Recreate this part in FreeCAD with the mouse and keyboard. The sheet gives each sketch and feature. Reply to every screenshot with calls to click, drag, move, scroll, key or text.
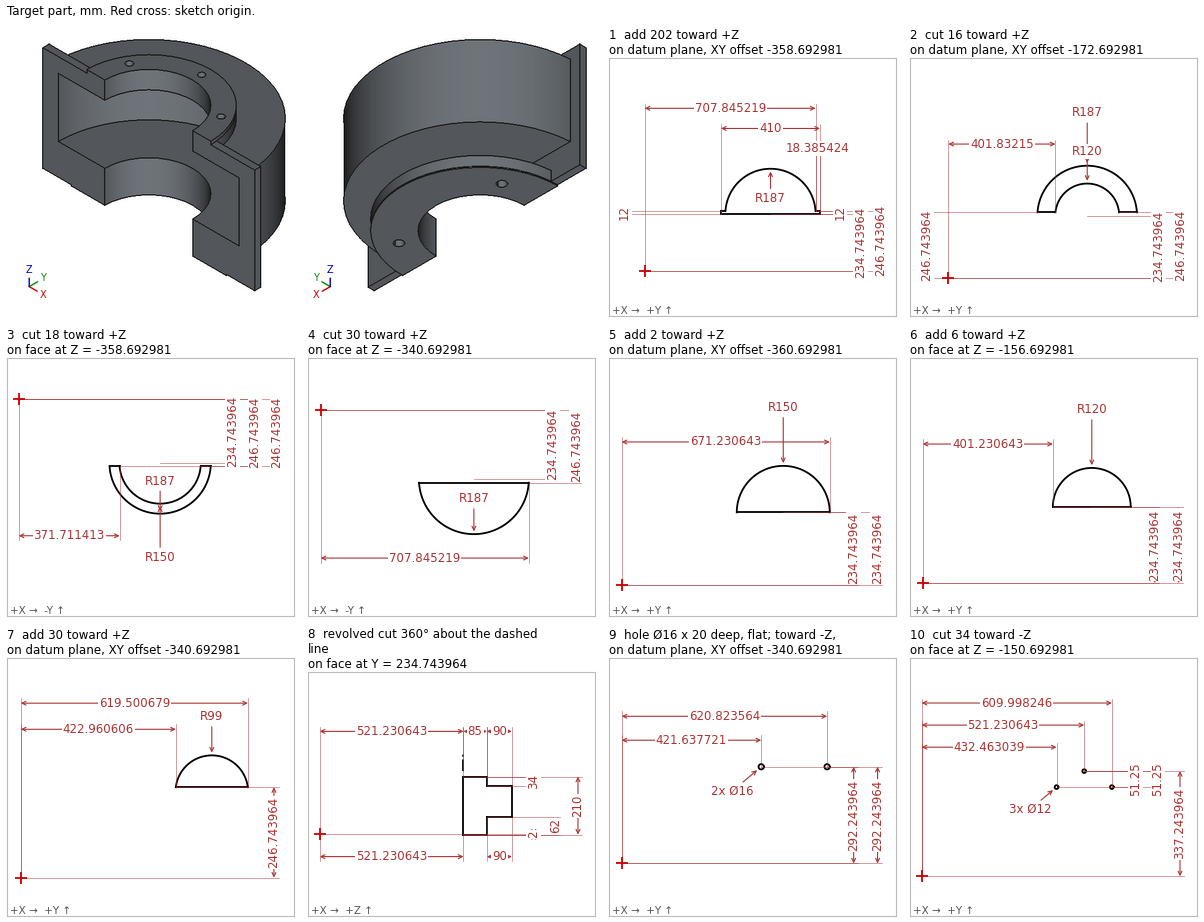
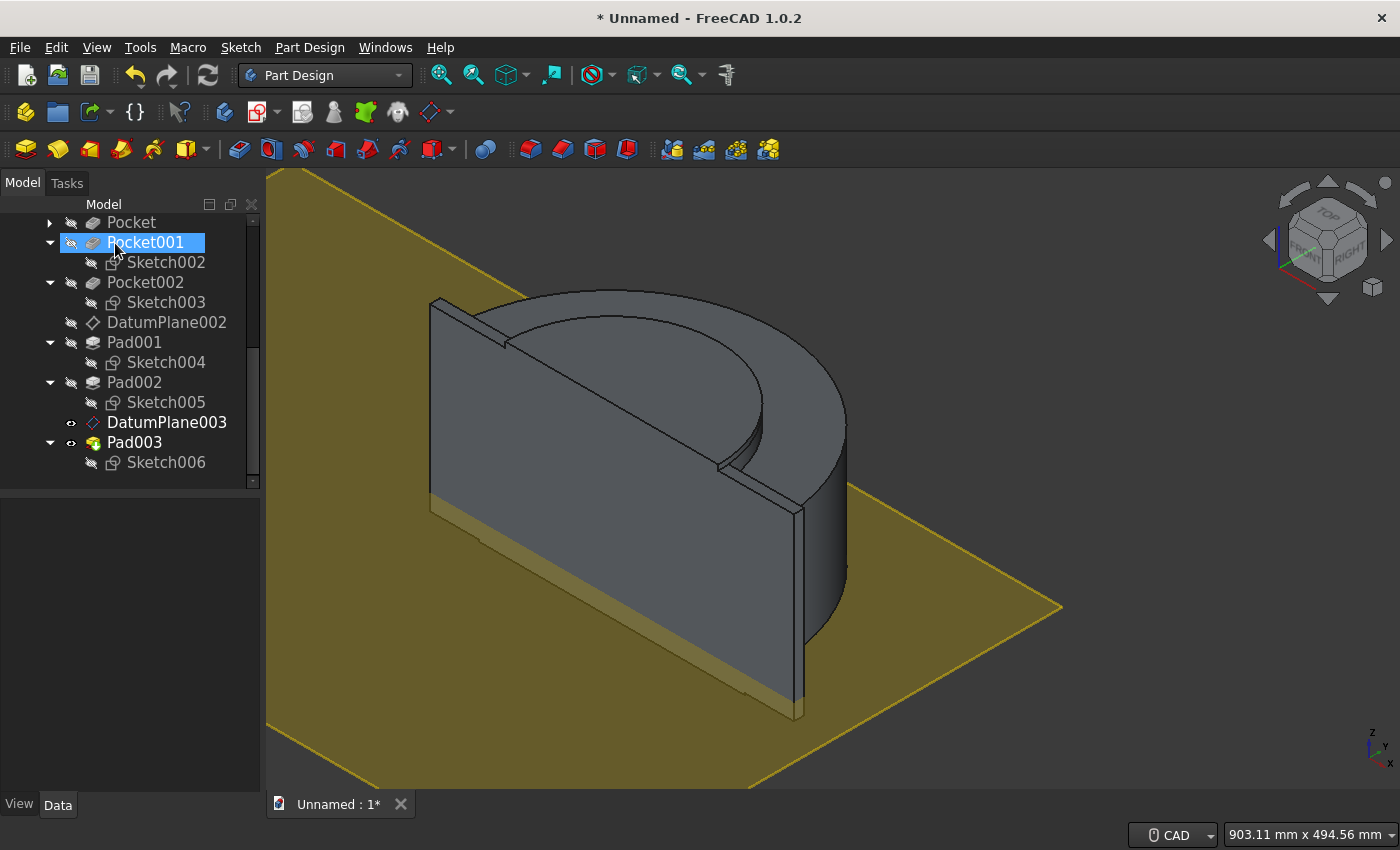
click(116, 423)
key(space)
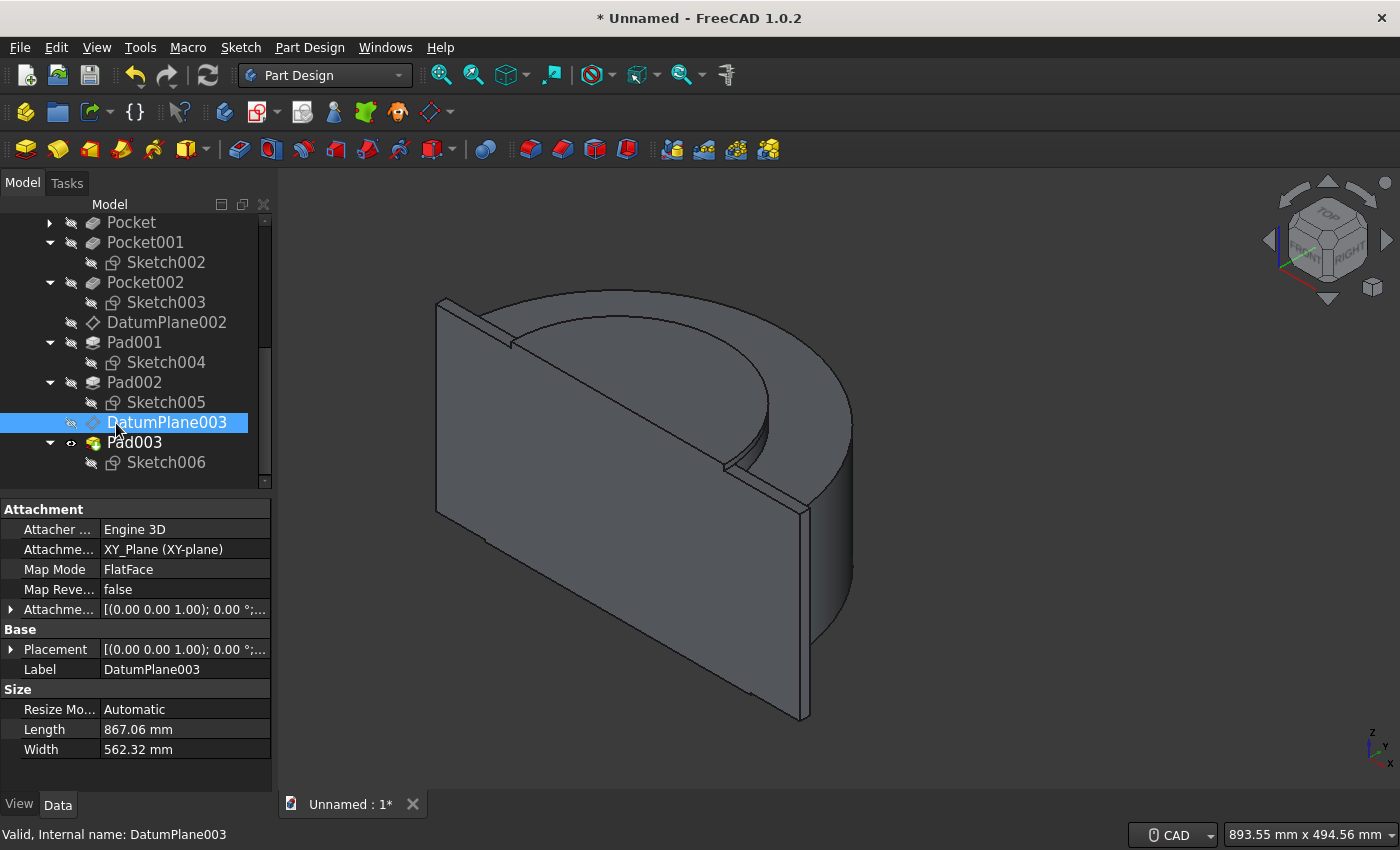
click(670, 540)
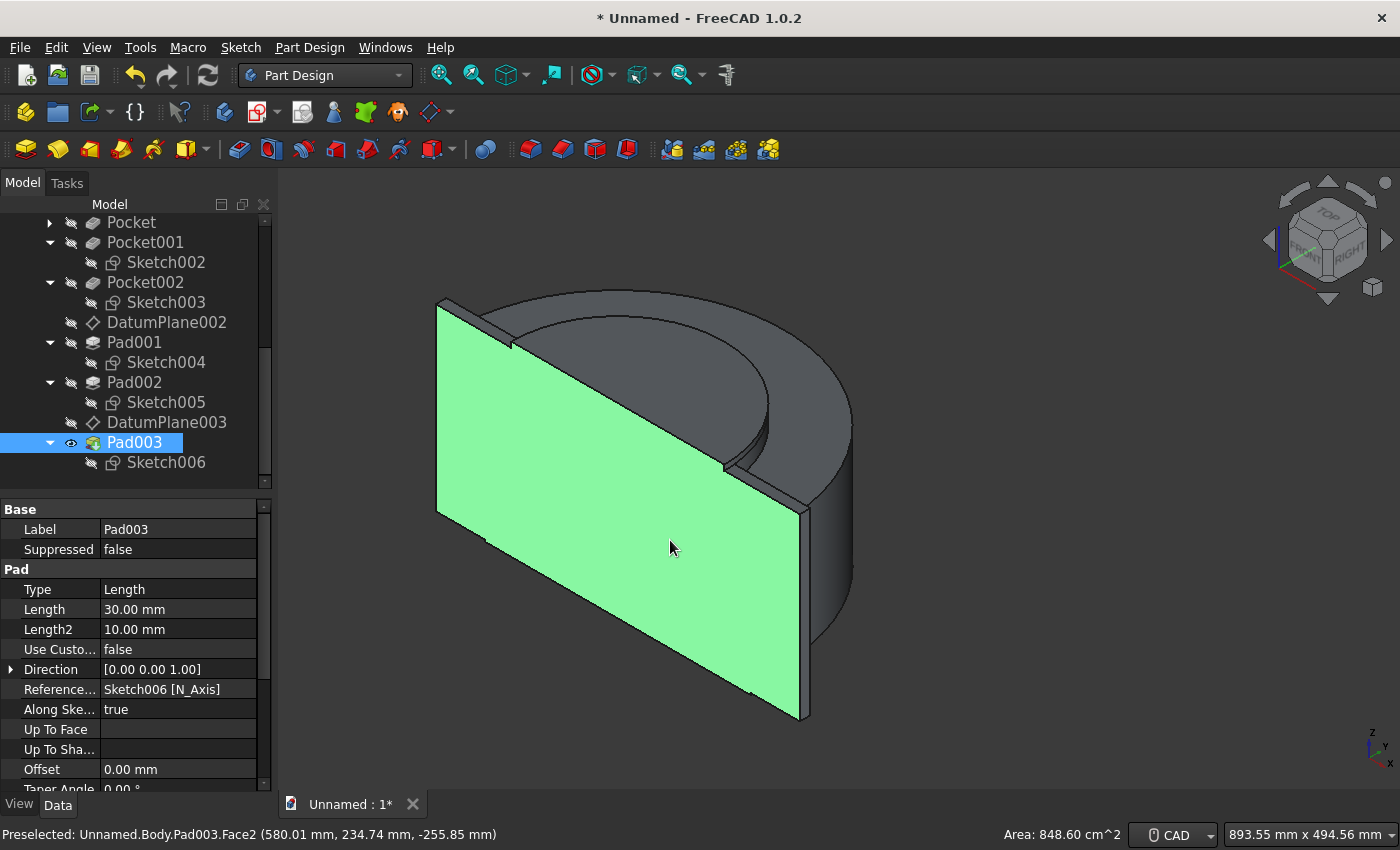
click(258, 112)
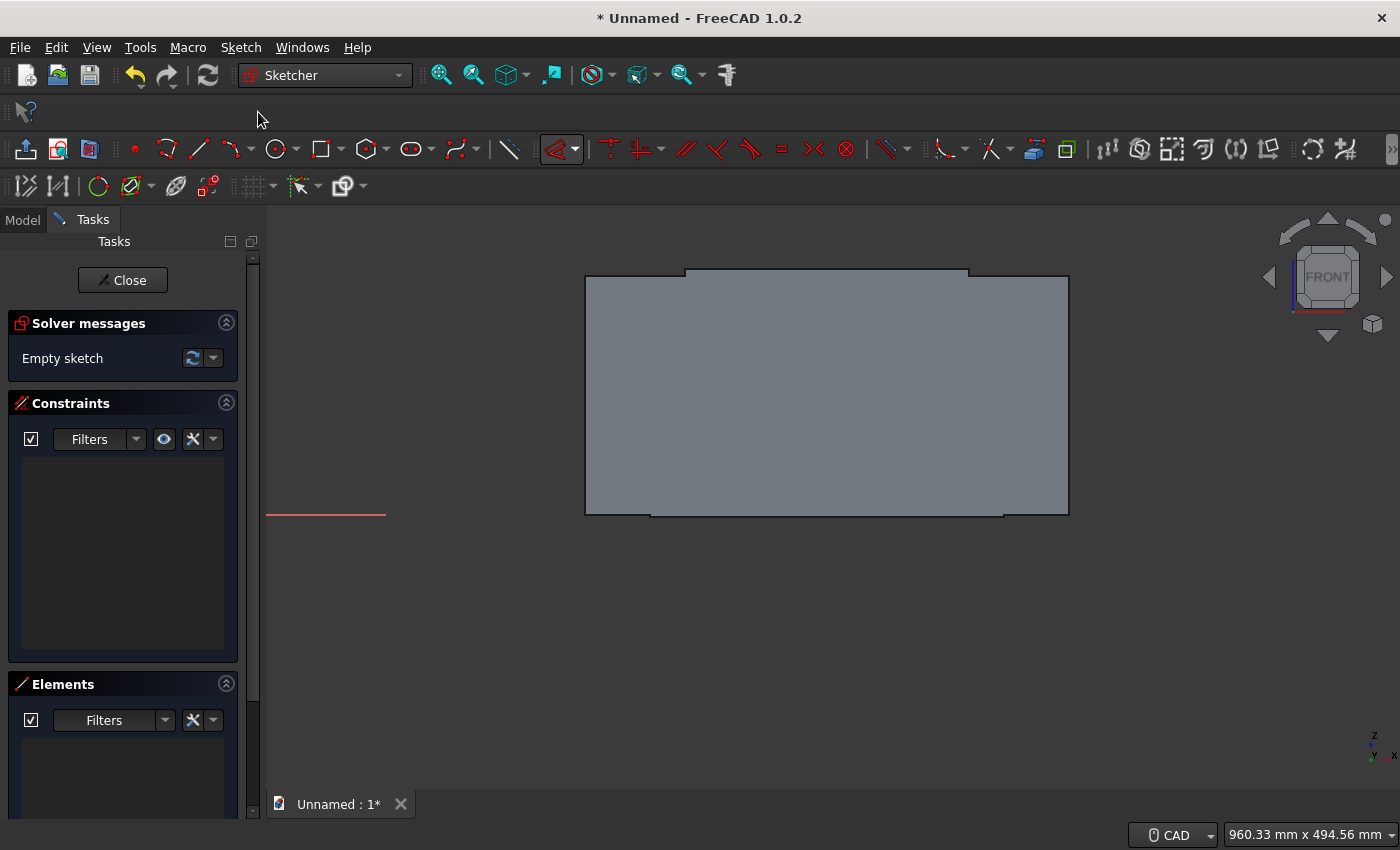
scroll(1235, 761, down, 1)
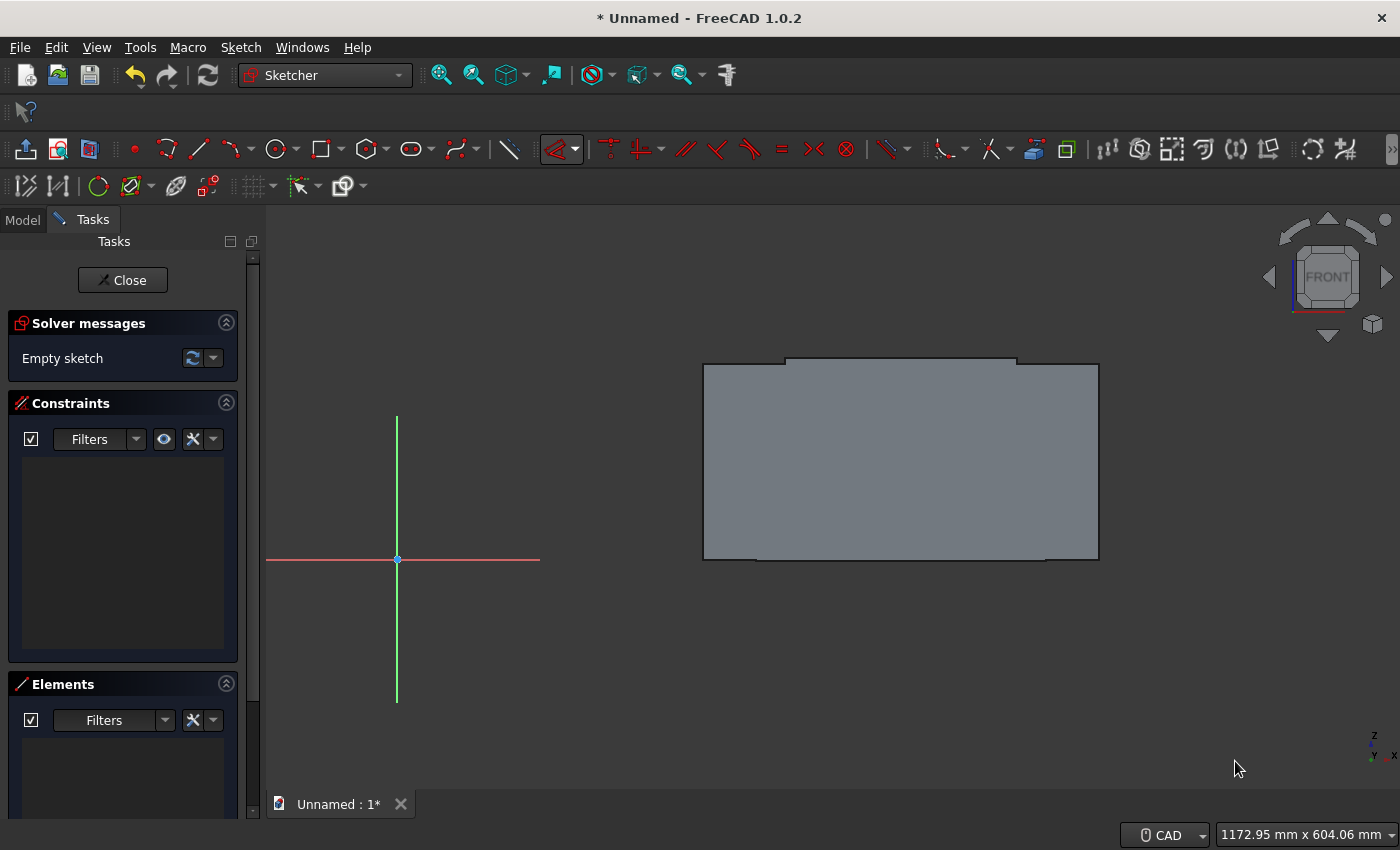
click(168, 150)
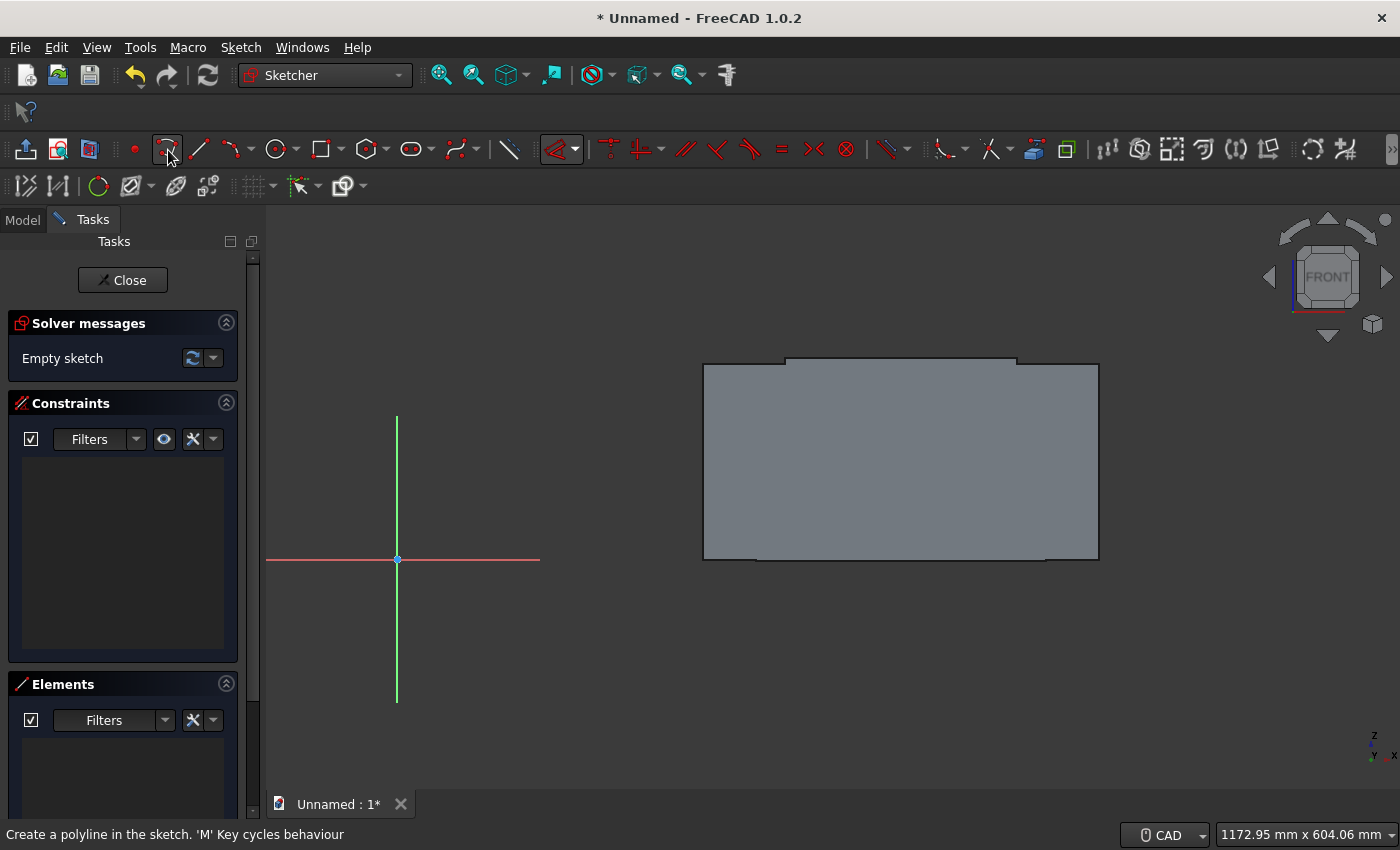
scroll(901, 561, up, 11)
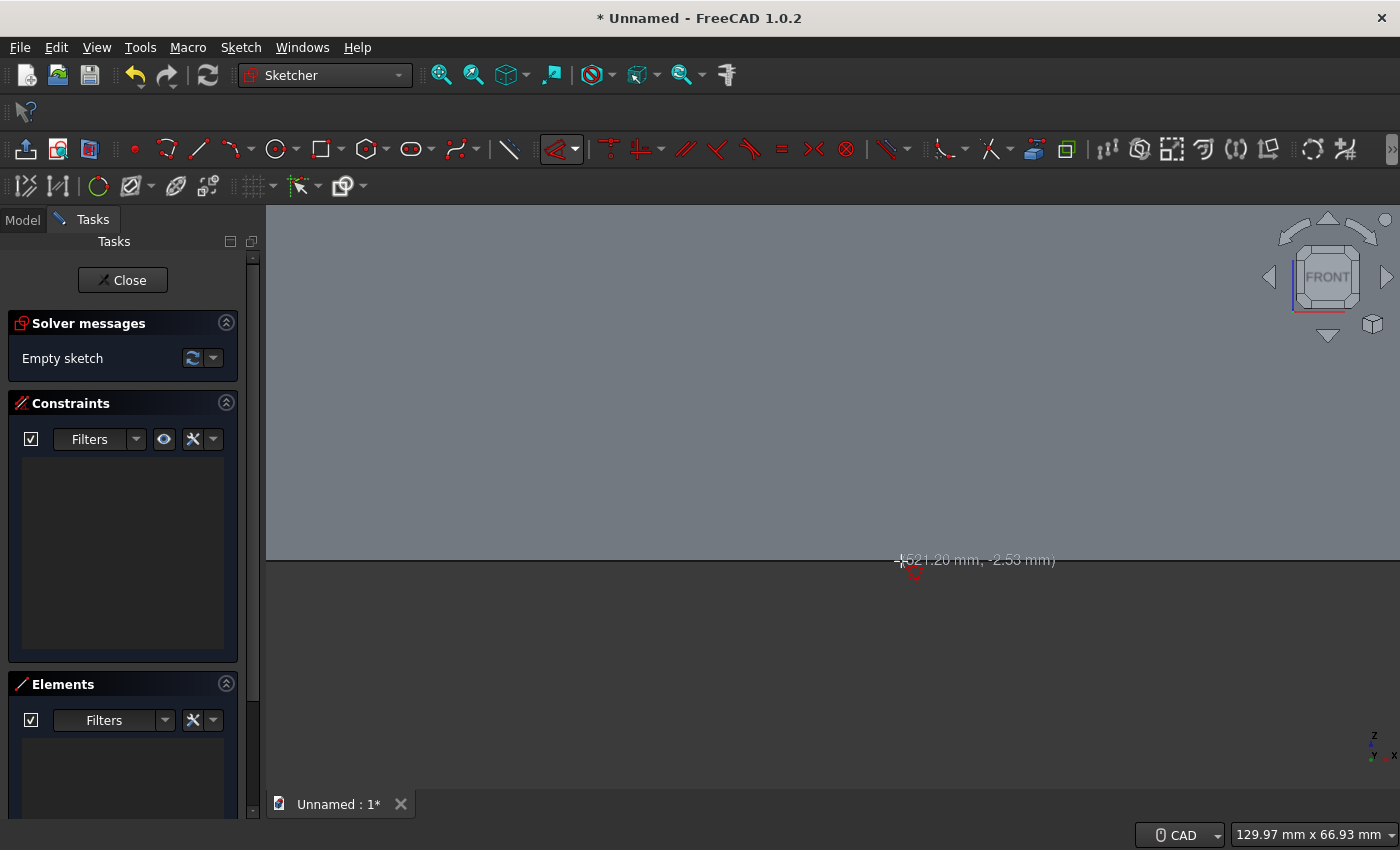
click(897, 561)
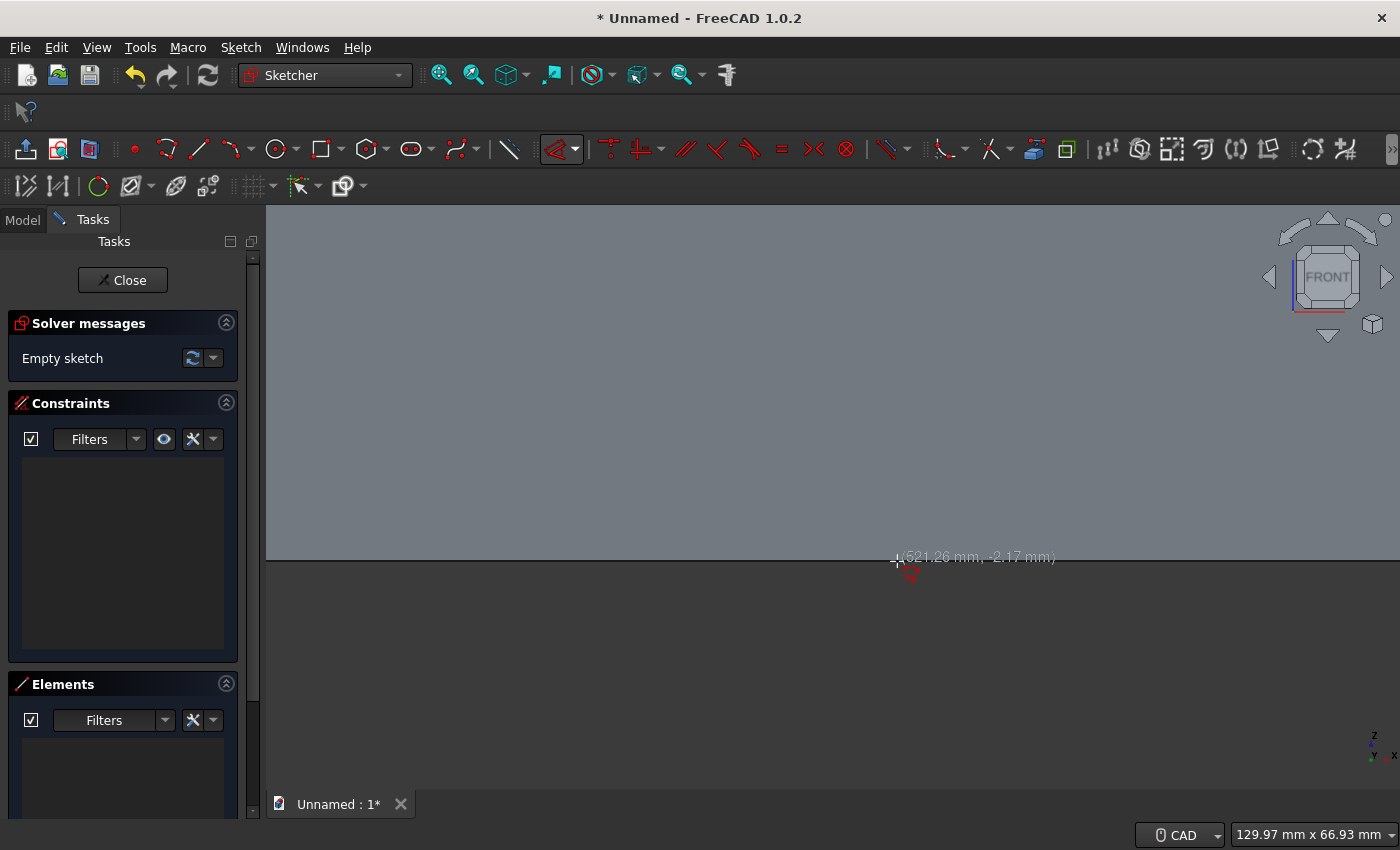
scroll(936, 649, down, 11)